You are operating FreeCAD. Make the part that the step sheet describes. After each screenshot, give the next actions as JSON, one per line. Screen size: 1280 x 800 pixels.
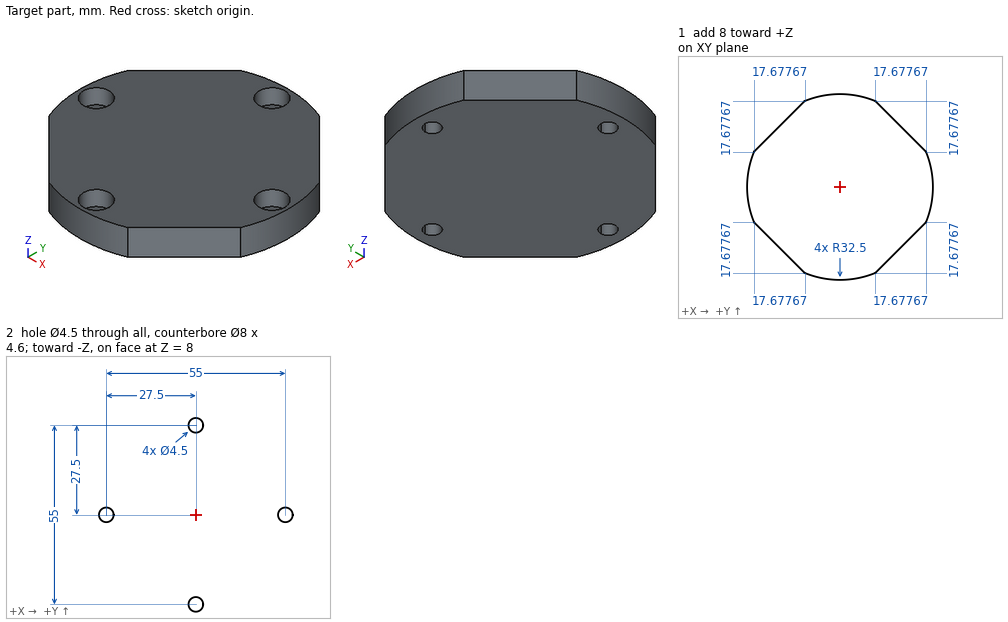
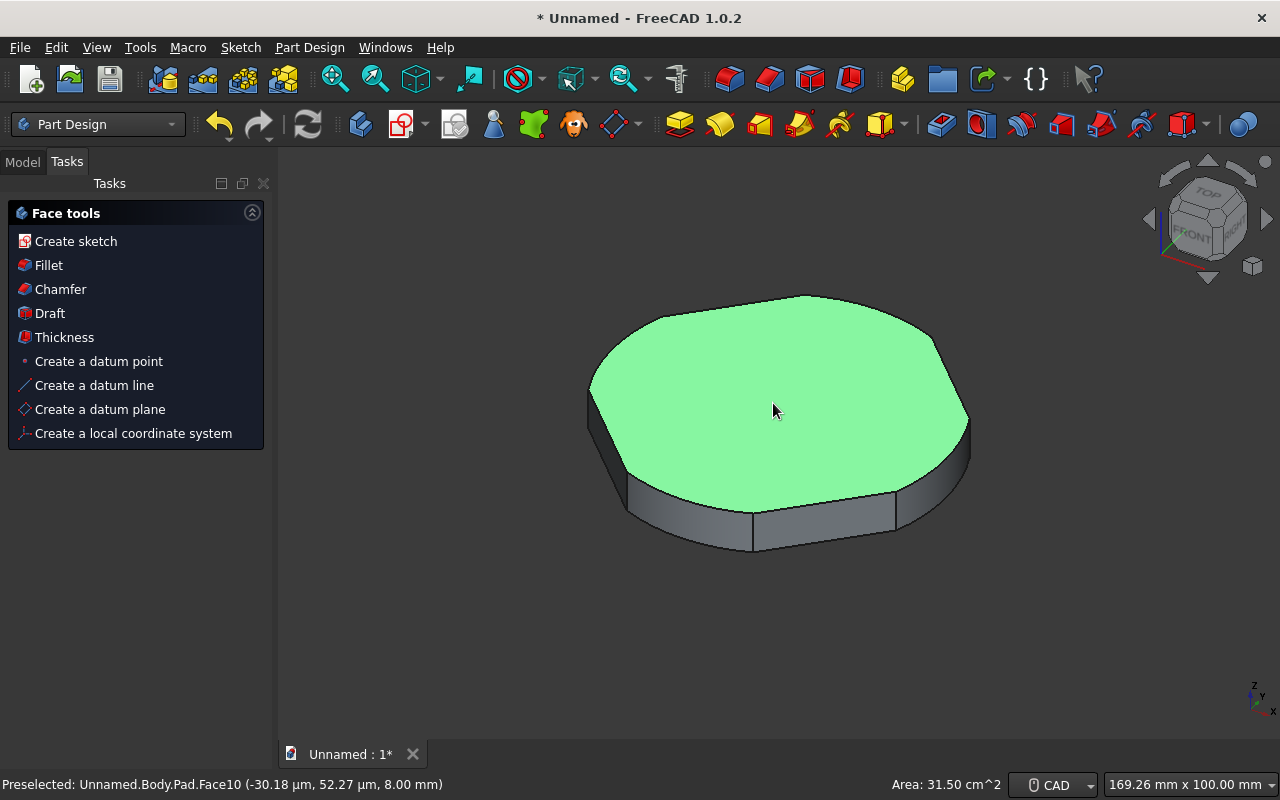
{"action": "left_click", "coordinate": [402, 124]}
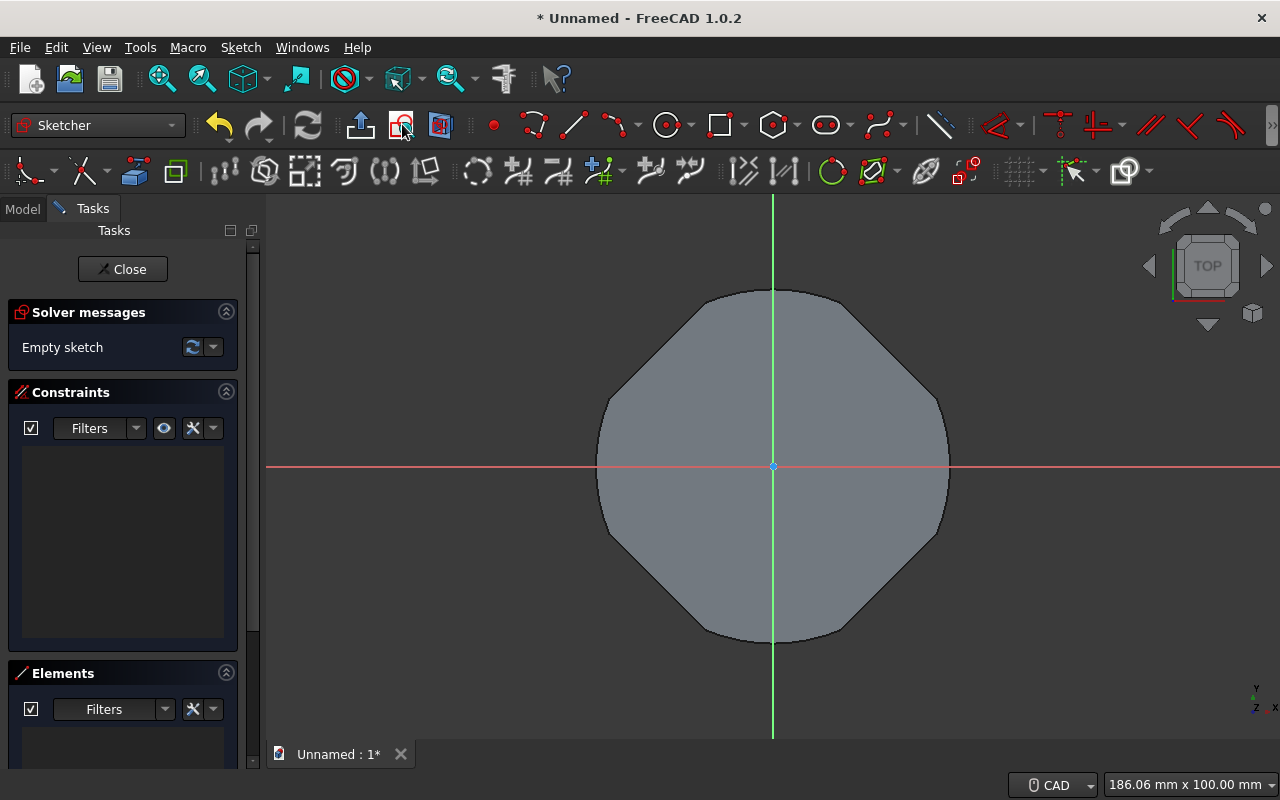
{"action": "left_click", "coordinate": [668, 126]}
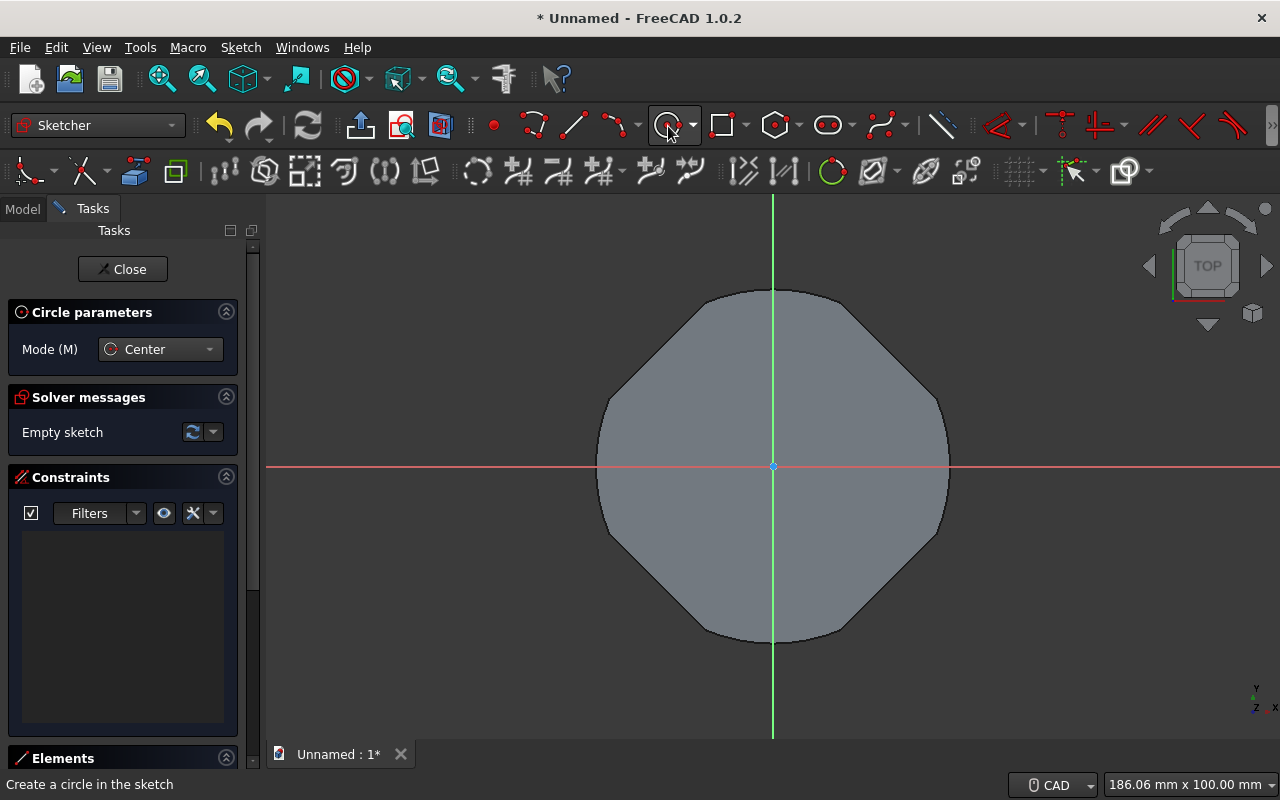
{"action": "scroll", "coordinate": [773, 317], "scroll_direction": "up", "scroll_amount": 4}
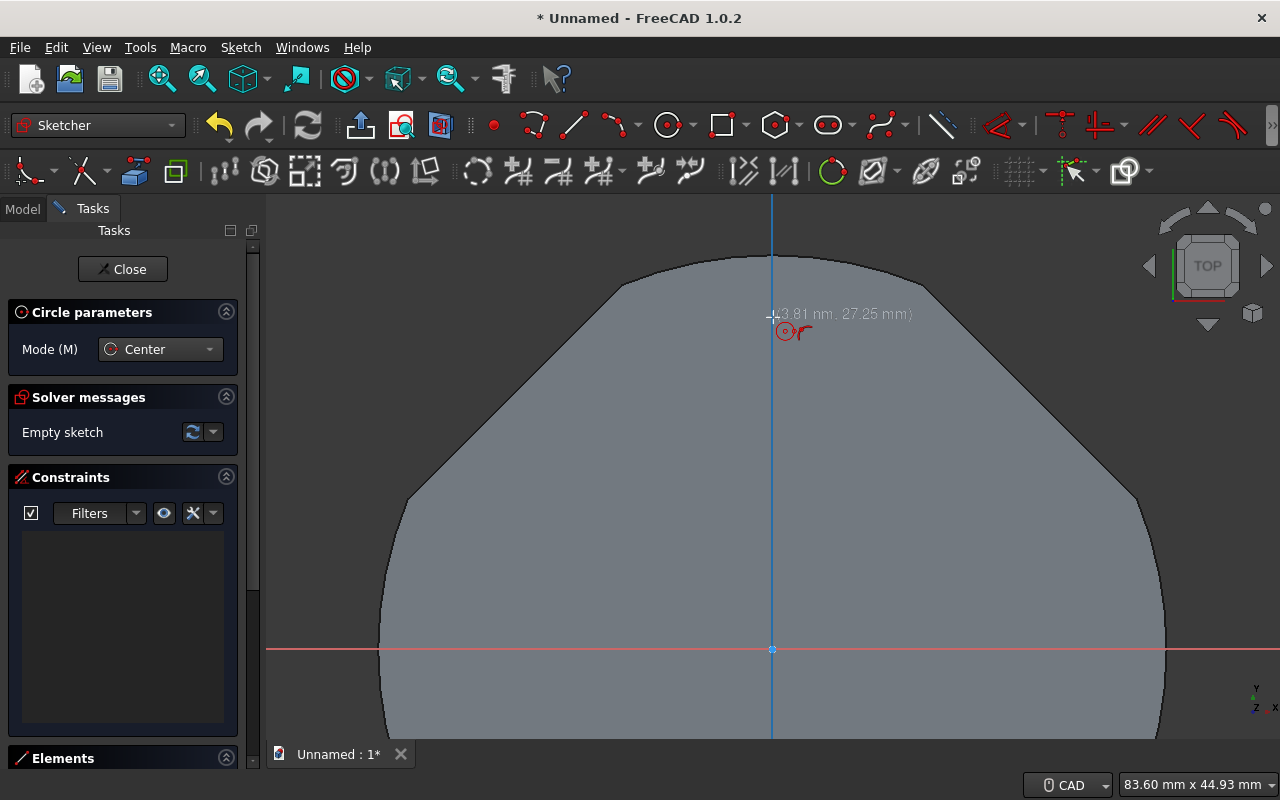
{"action": "left_click", "coordinate": [772, 316]}
{"action": "left_click", "coordinate": [792, 297]}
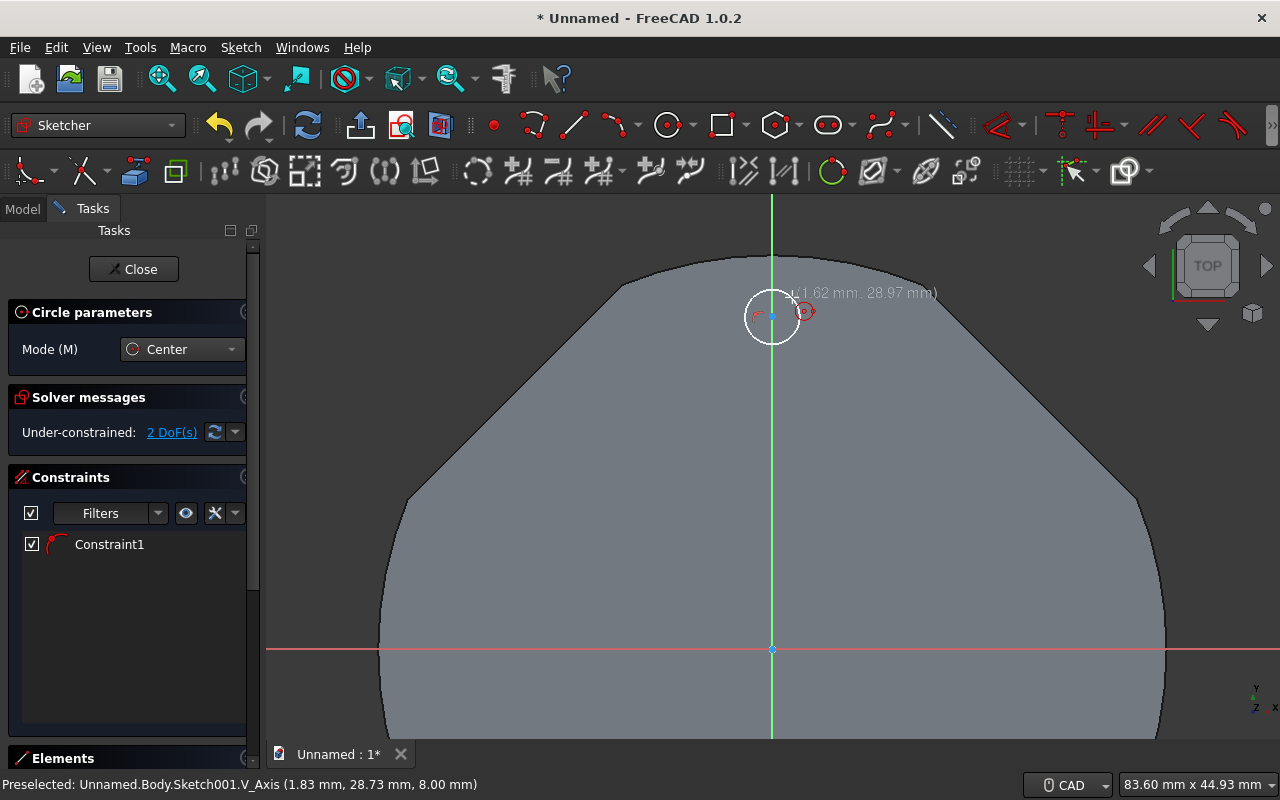
{"action": "left_click", "coordinate": [439, 649]}
{"action": "left_click", "coordinate": [458, 630]}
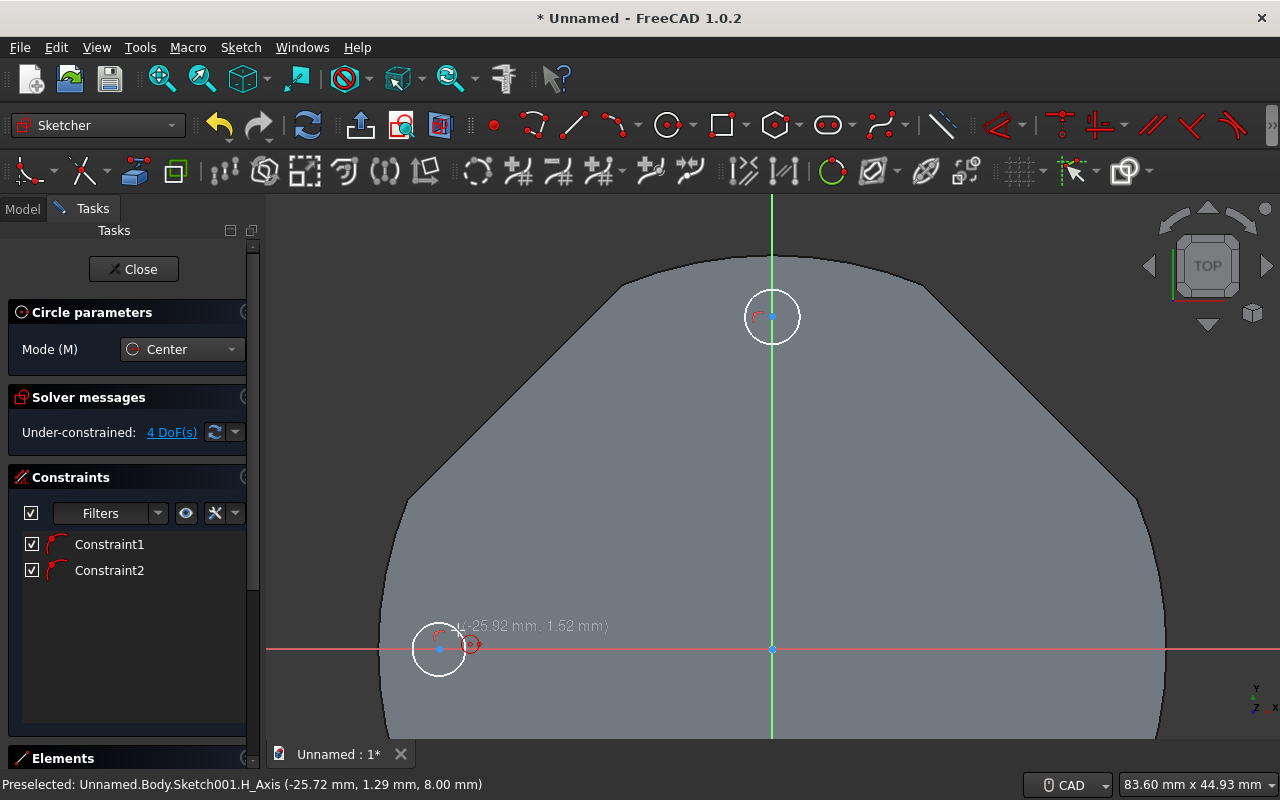
{"action": "scroll", "coordinate": [649, 317], "scroll_direction": "down", "scroll_amount": 4}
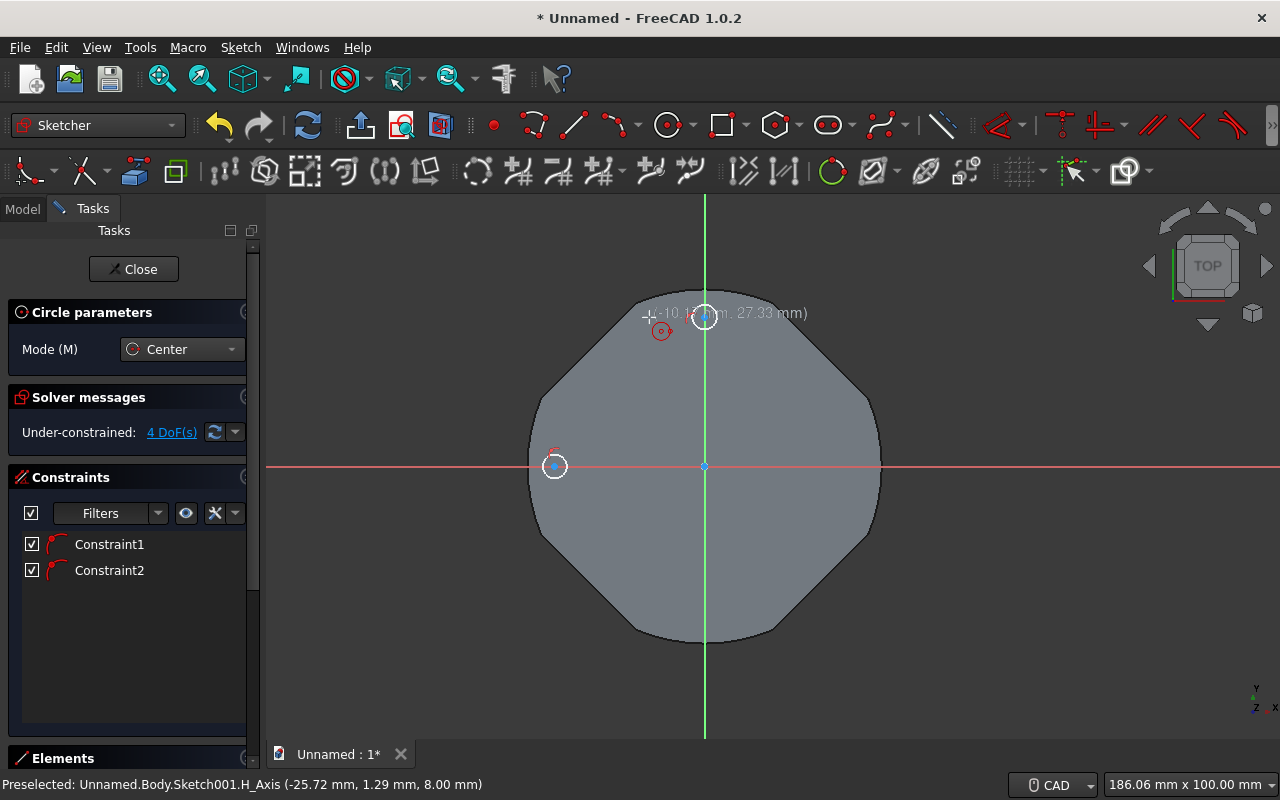
{"action": "scroll", "coordinate": [705, 616], "scroll_direction": "up", "scroll_amount": 4}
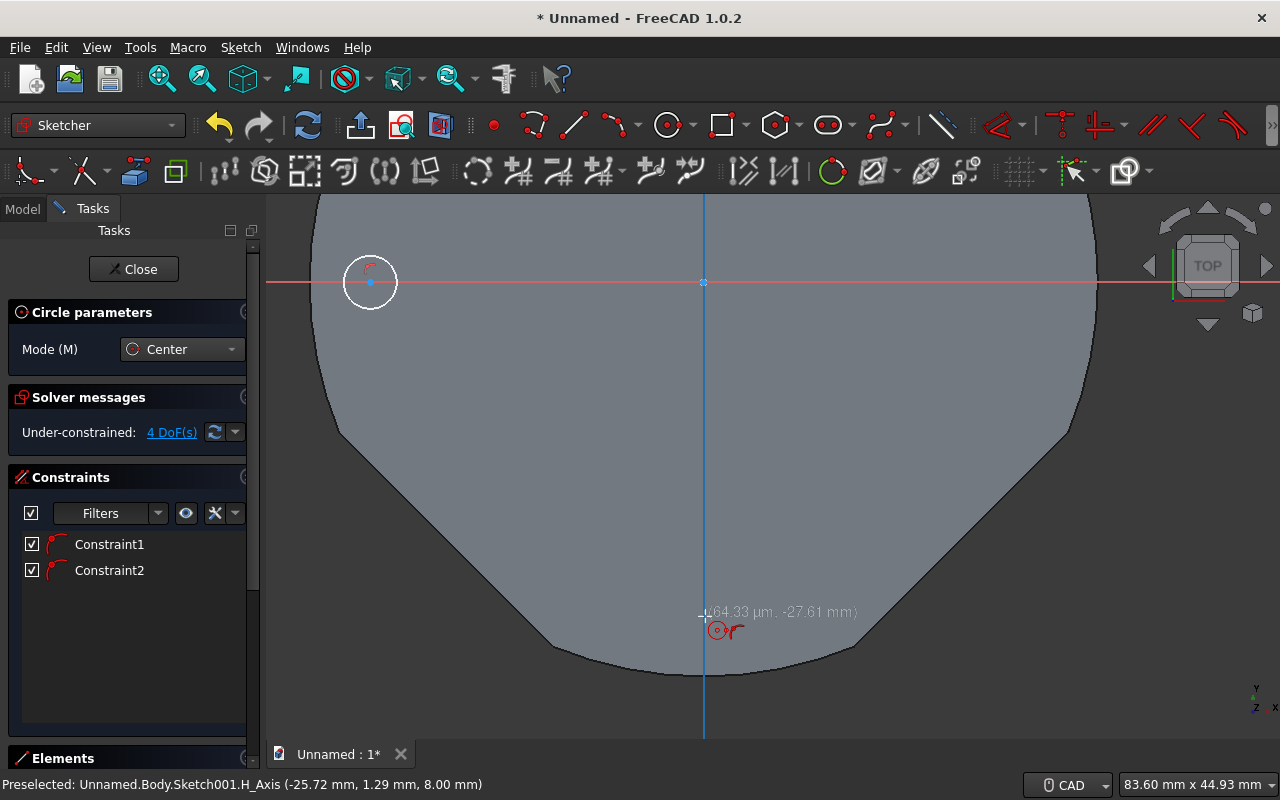
{"action": "left_click", "coordinate": [704, 616]}
{"action": "left_click", "coordinate": [723, 597]}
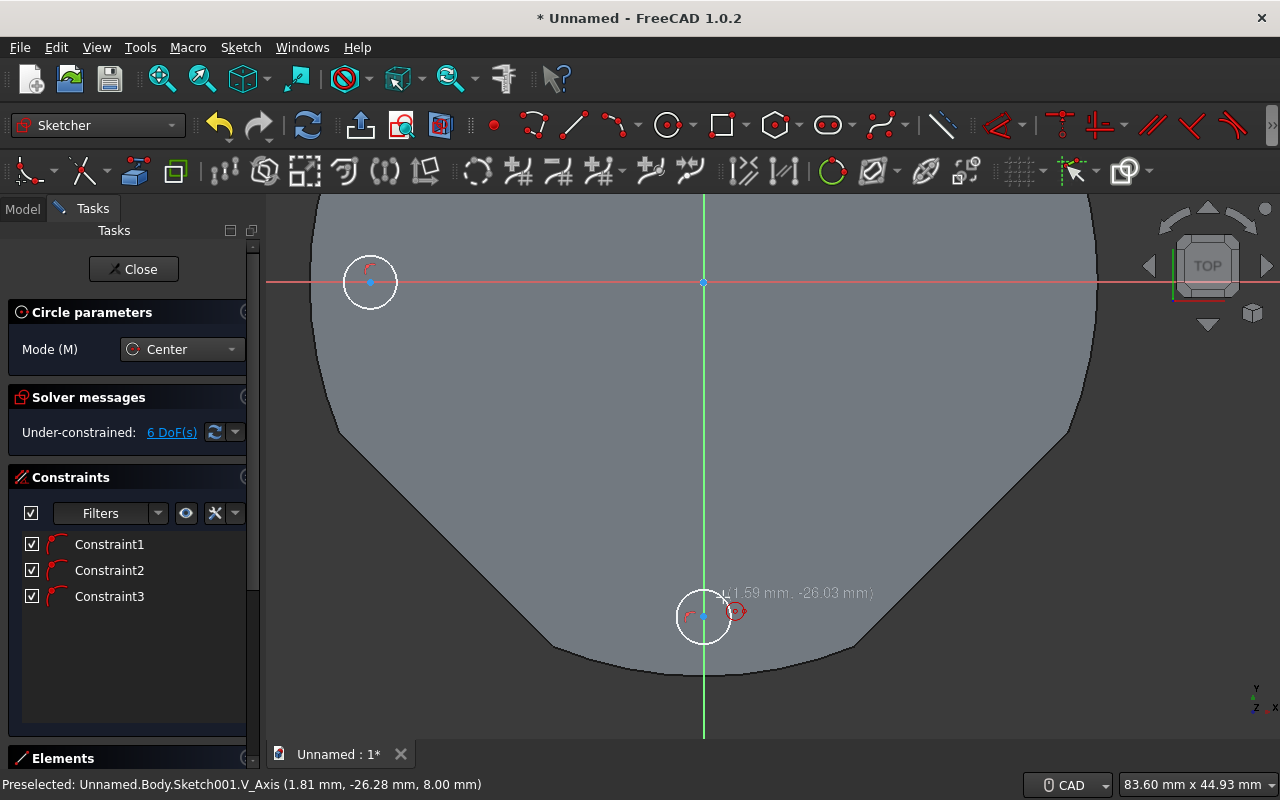
{"action": "left_click", "coordinate": [1037, 282]}
{"action": "left_click", "coordinate": [1057, 263]}
{"action": "key", "text": "Escape"}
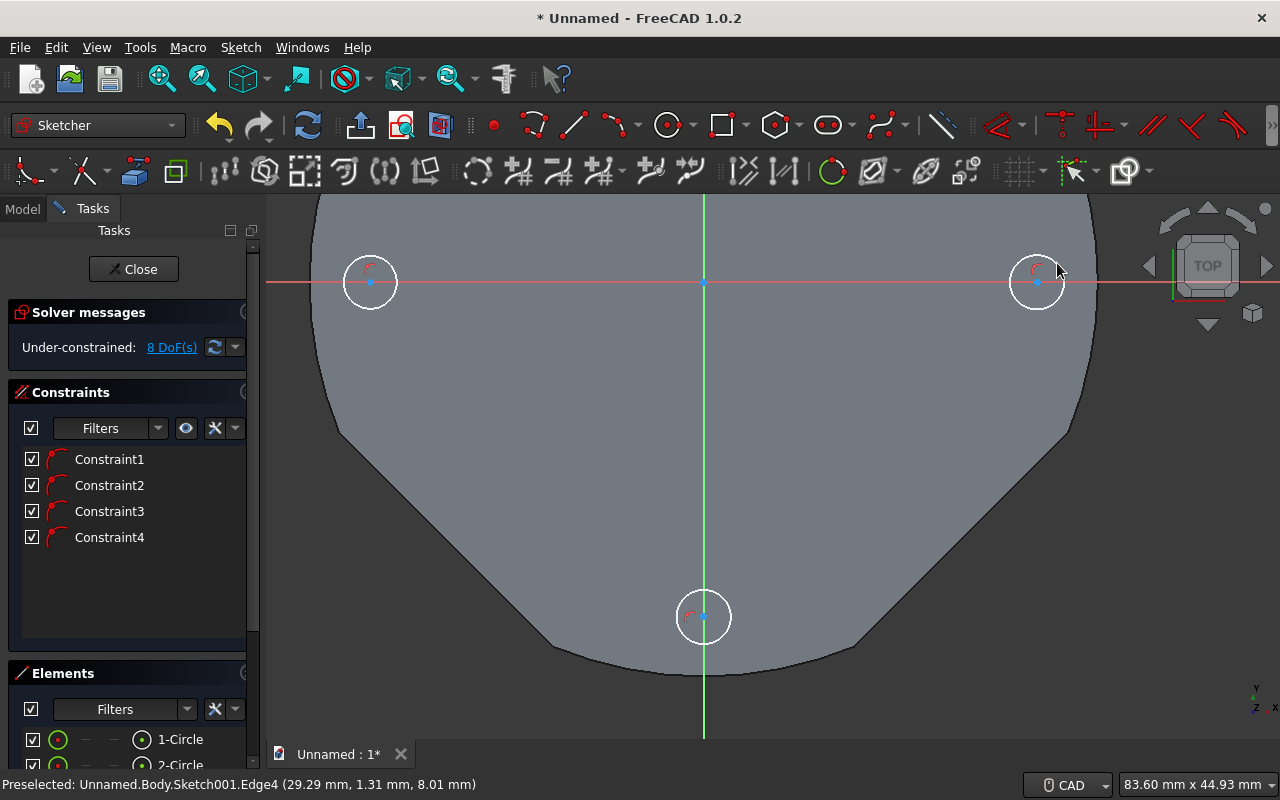
{"action": "scroll", "coordinate": [705, 617], "scroll_direction": "down", "scroll_amount": 4}